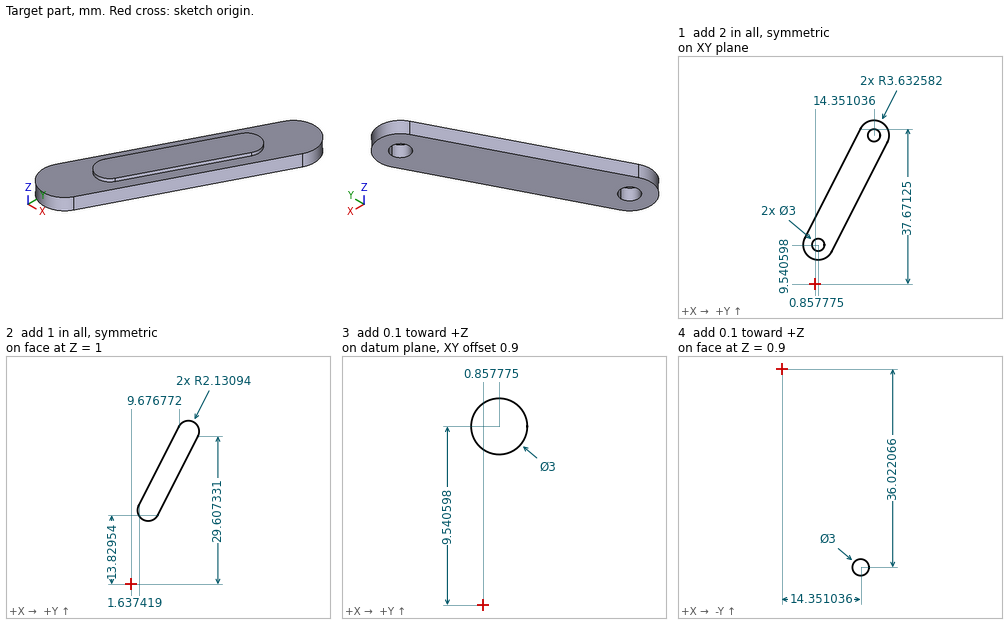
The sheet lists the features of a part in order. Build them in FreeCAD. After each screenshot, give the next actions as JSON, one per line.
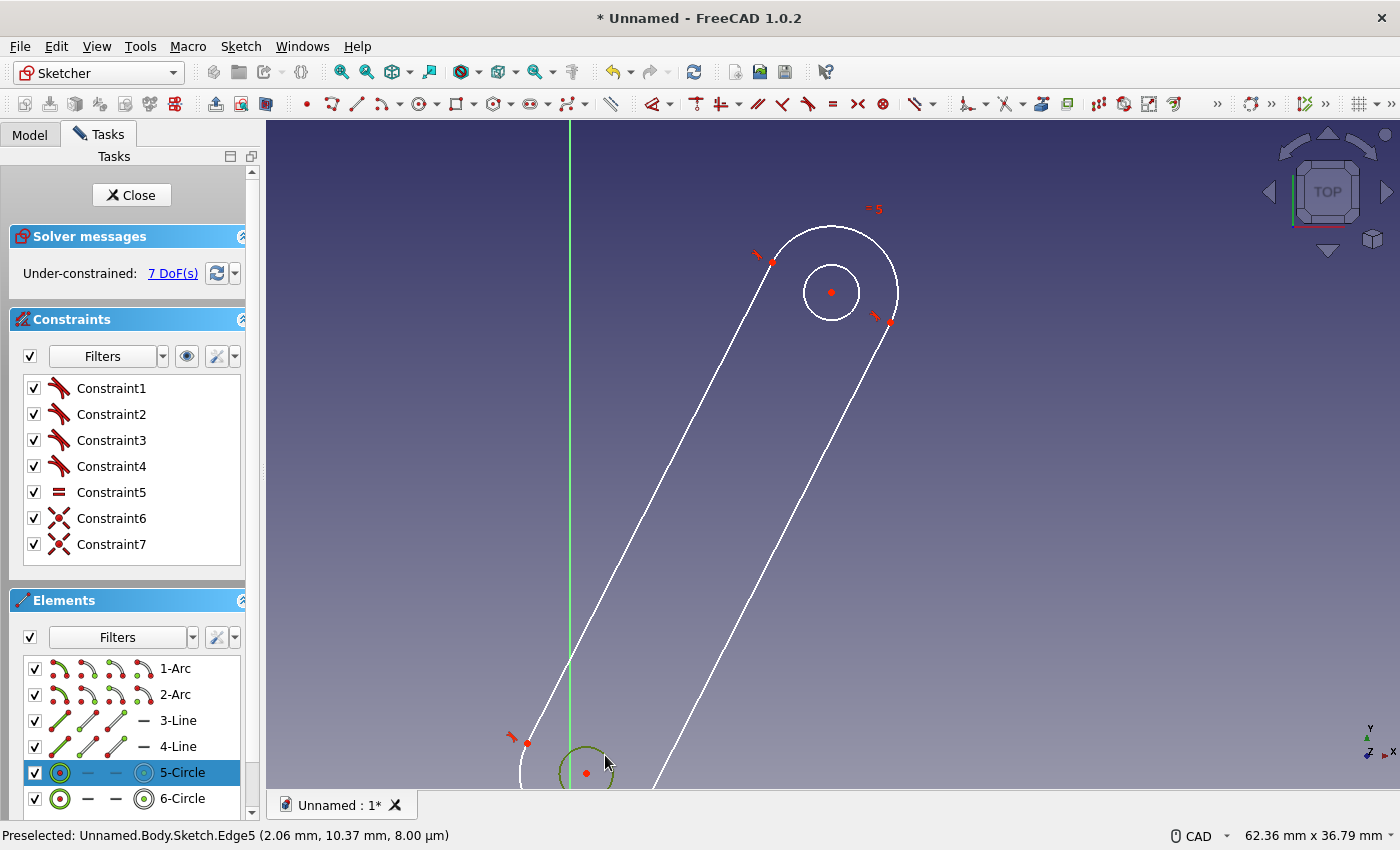
{"action": "left_click", "coordinate": [851, 273]}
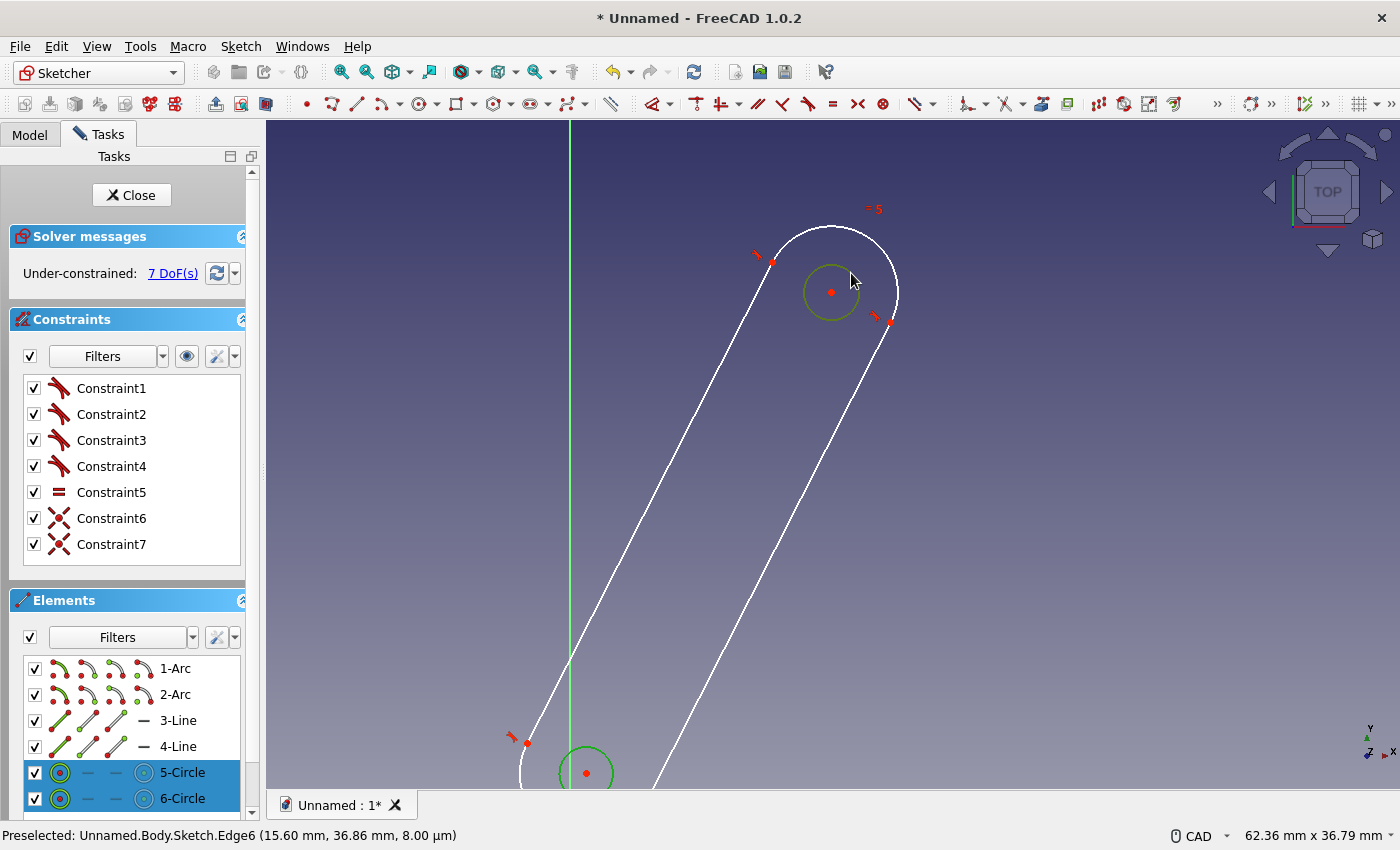
{"action": "key", "text": "e"}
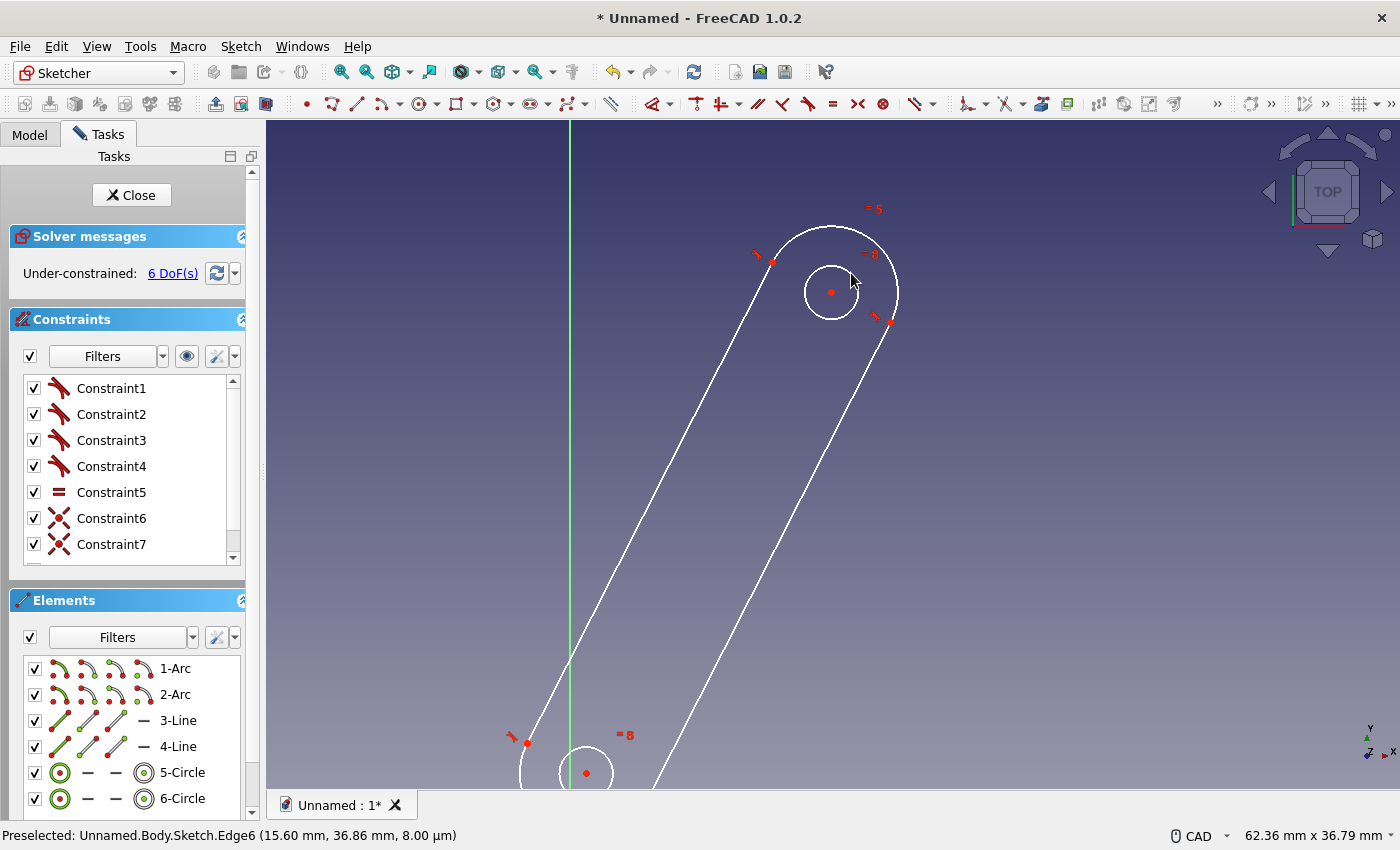
{"action": "scroll", "coordinate": [833, 290], "scroll_direction": "down", "scroll_amount": 3}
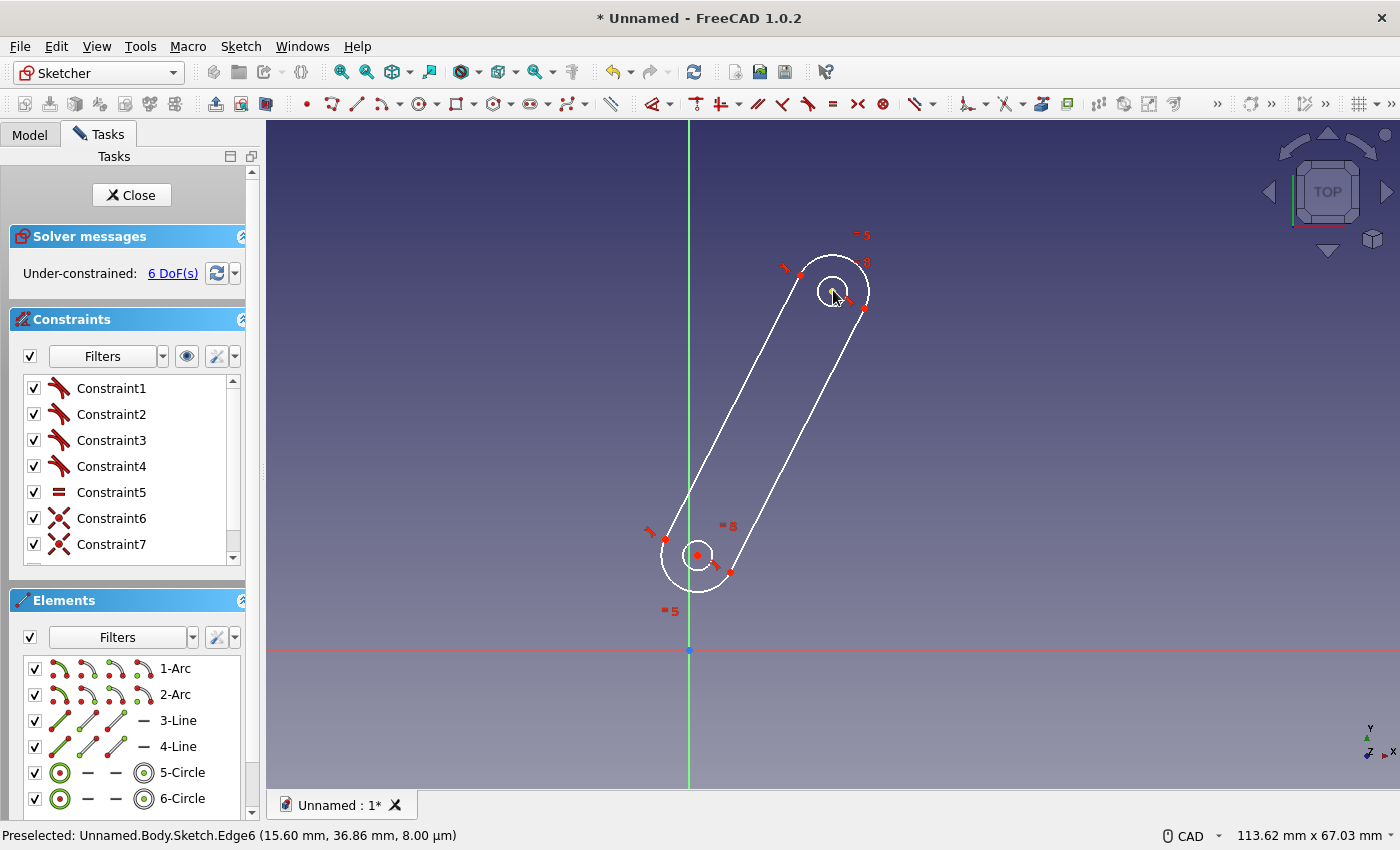
{"action": "left_click", "coordinate": [665, 572]}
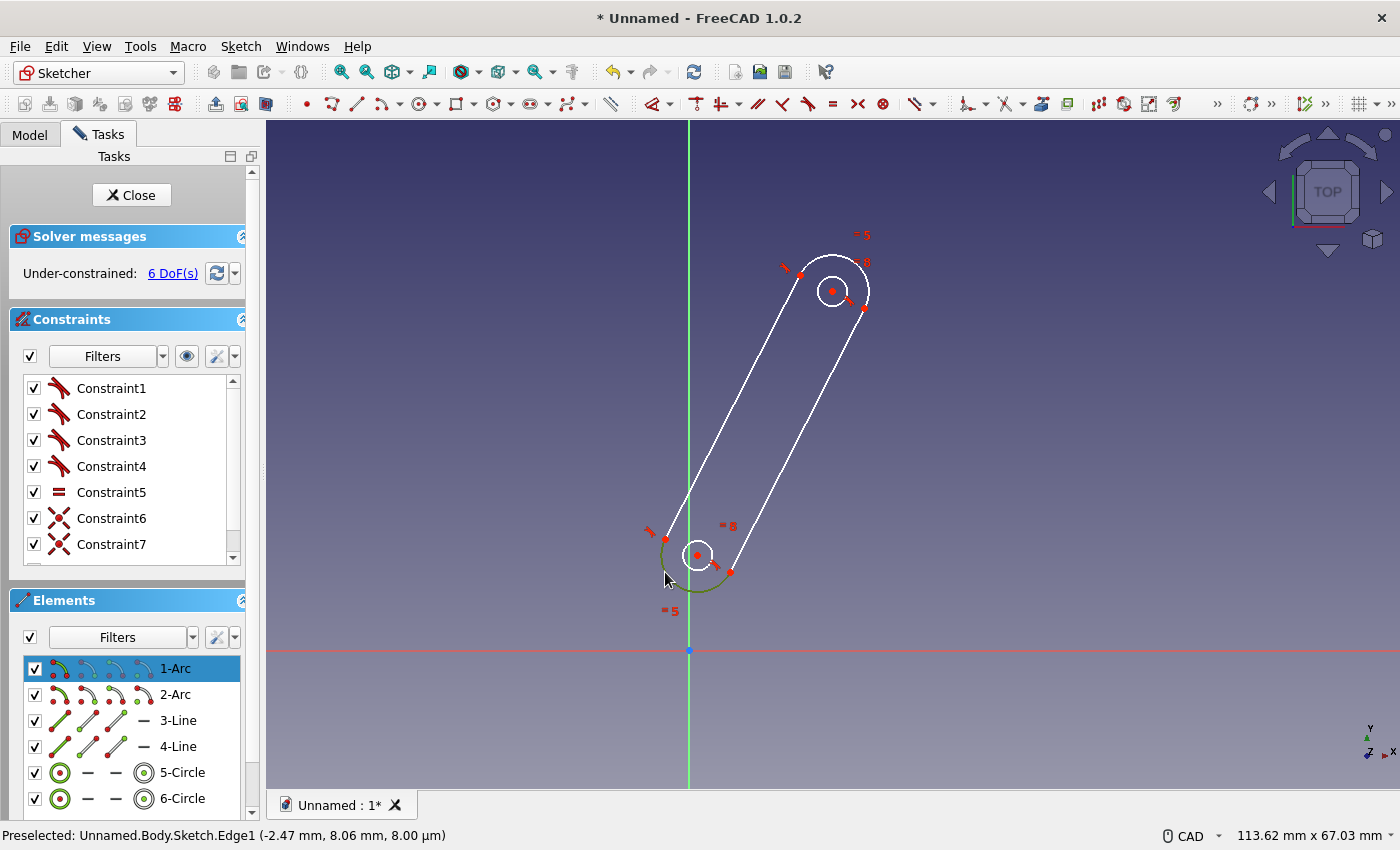
{"action": "key", "text": "k r"}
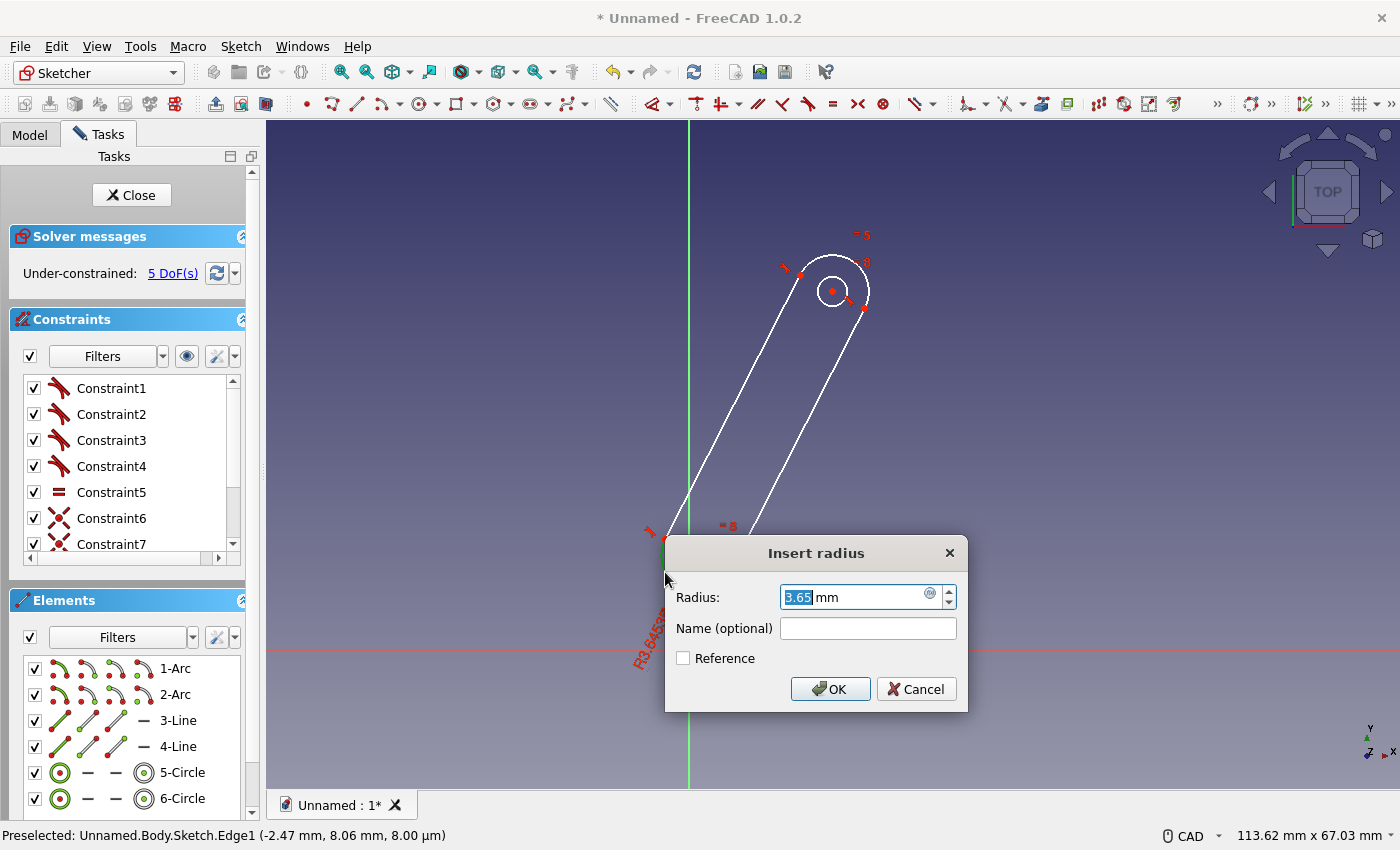
{"action": "type", "text": "3.632582"}
{"action": "key", "text": "Return"}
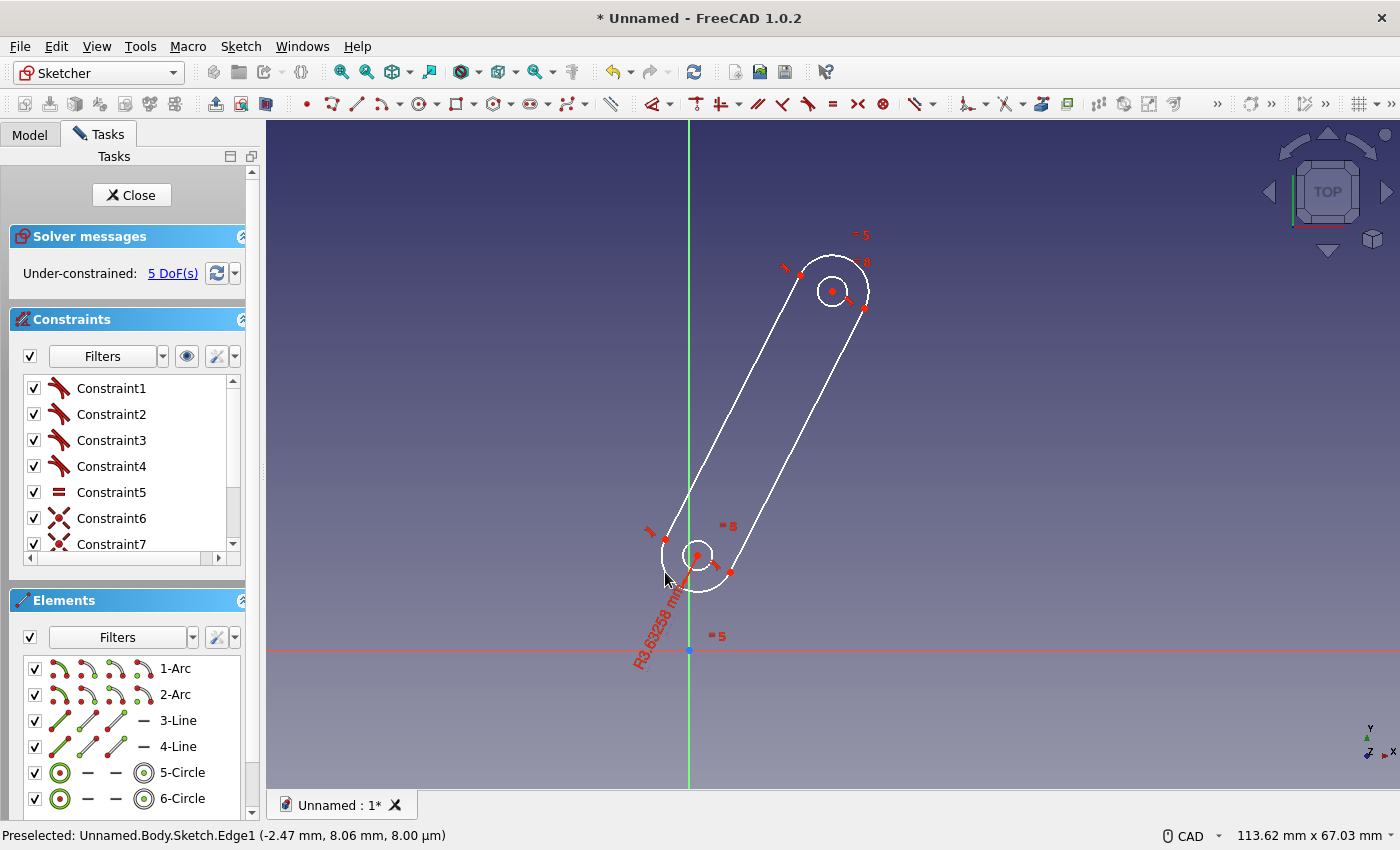
{"action": "scroll", "coordinate": [708, 545], "scroll_direction": "up", "scroll_amount": 2}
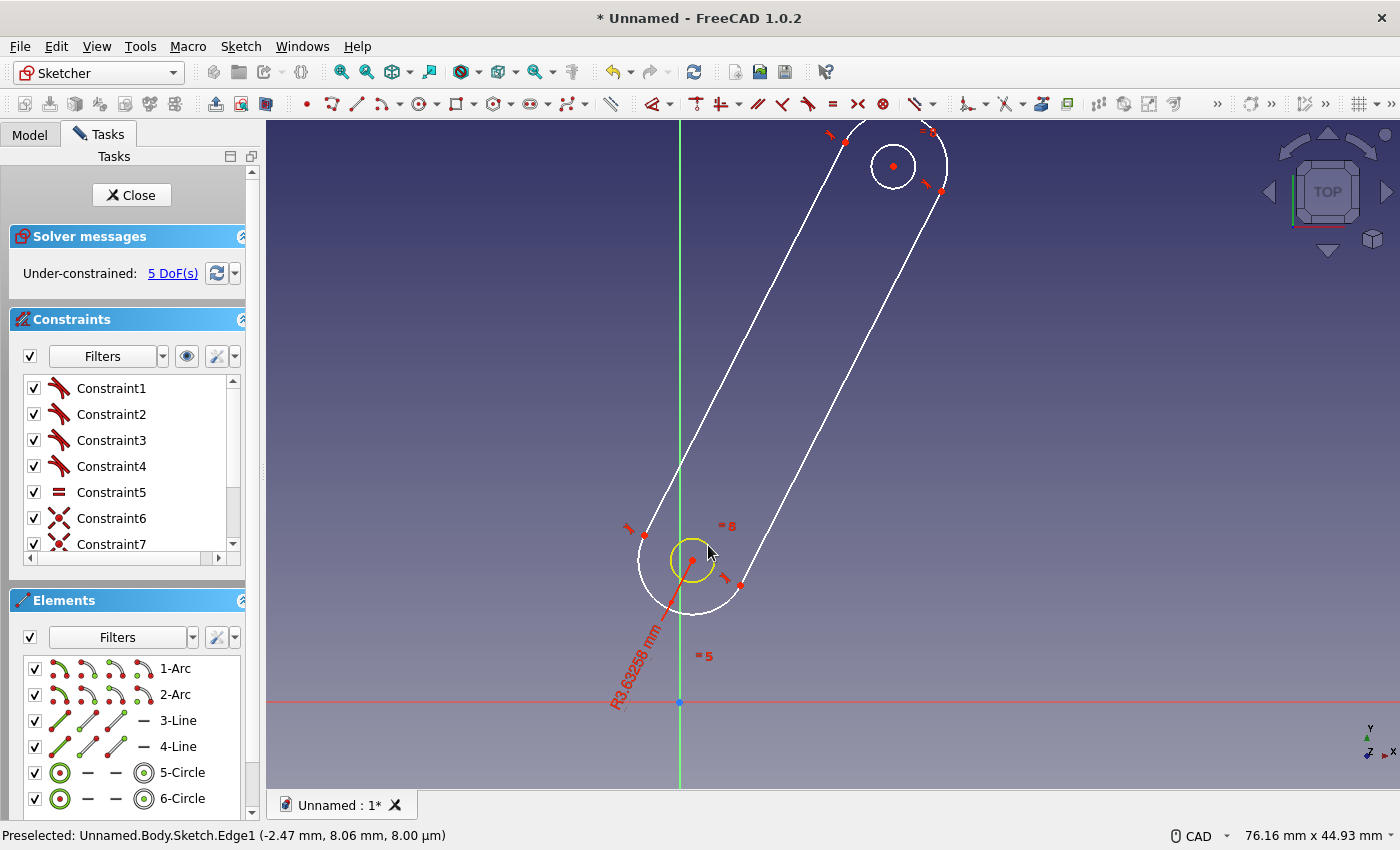
{"action": "left_click", "coordinate": [708, 545]}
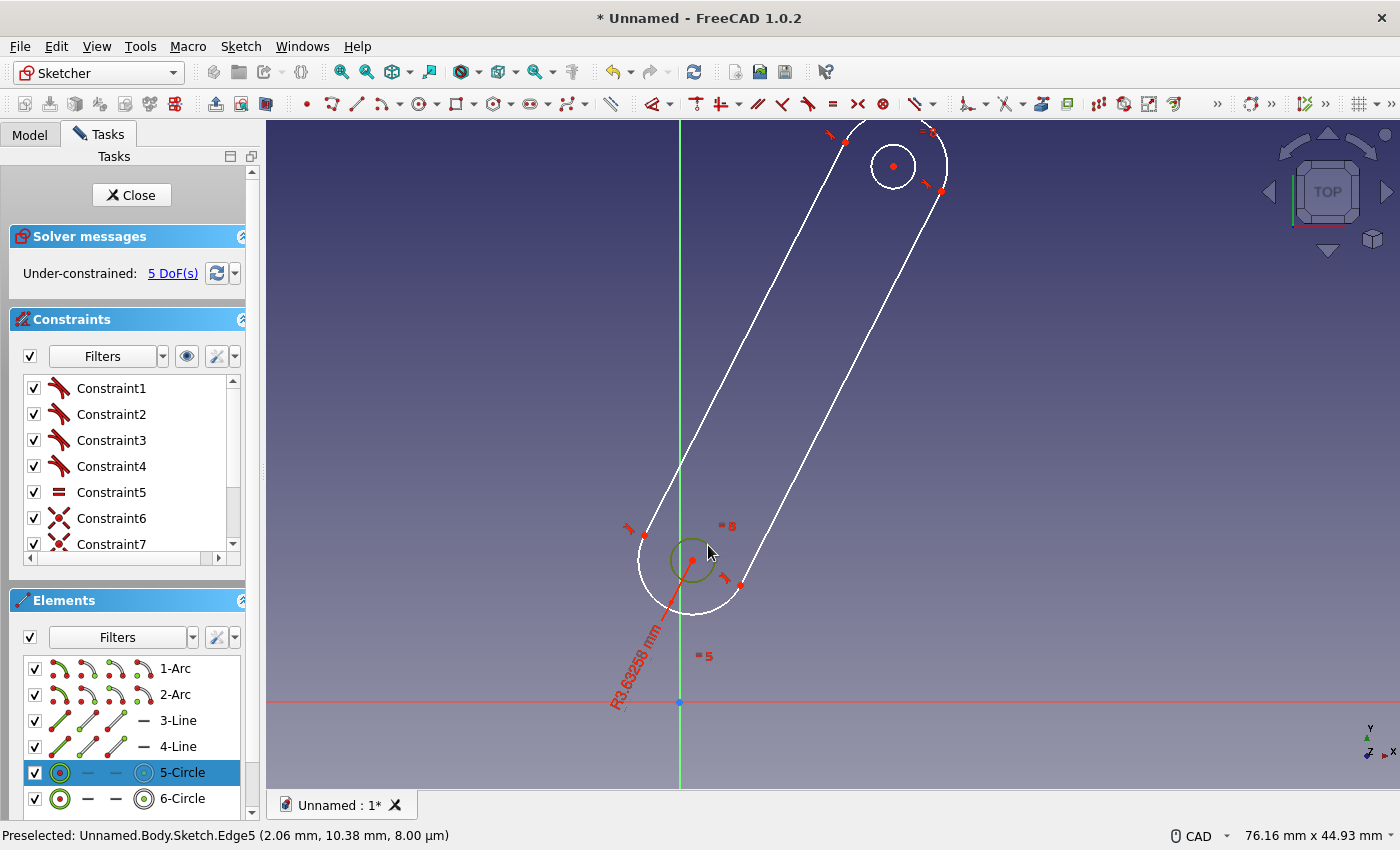
{"action": "left_click", "coordinate": [670, 104]}